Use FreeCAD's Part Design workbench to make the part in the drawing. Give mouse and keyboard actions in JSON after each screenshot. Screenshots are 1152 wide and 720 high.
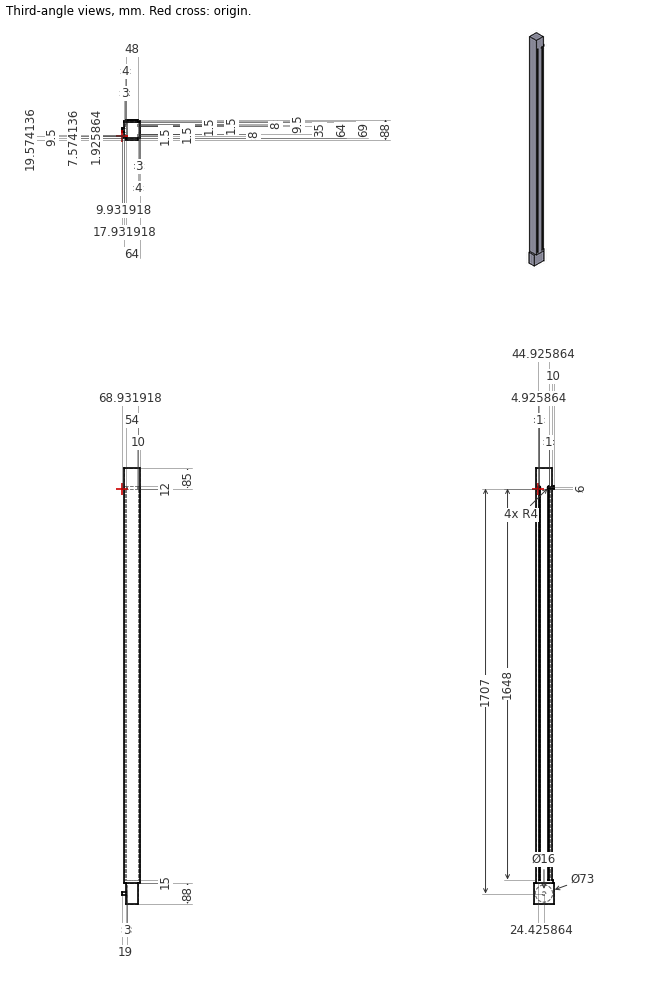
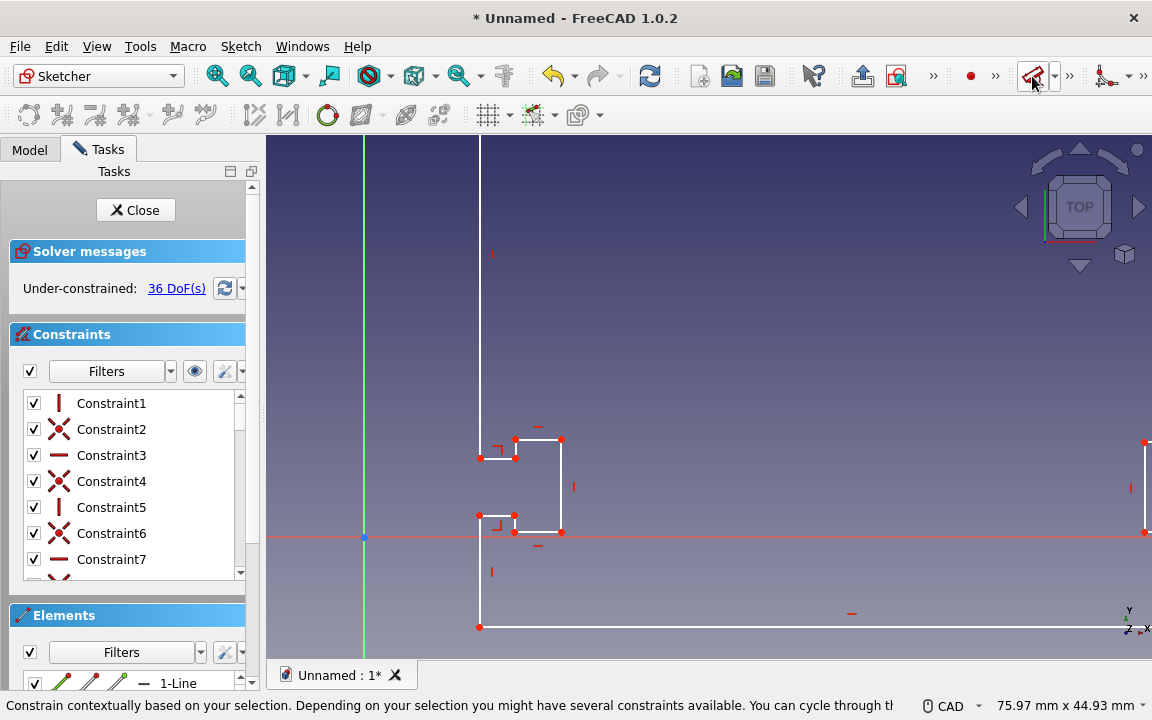
{"action": "scroll", "coordinate": [514, 515], "scroll_direction": "down", "scroll_amount": 4}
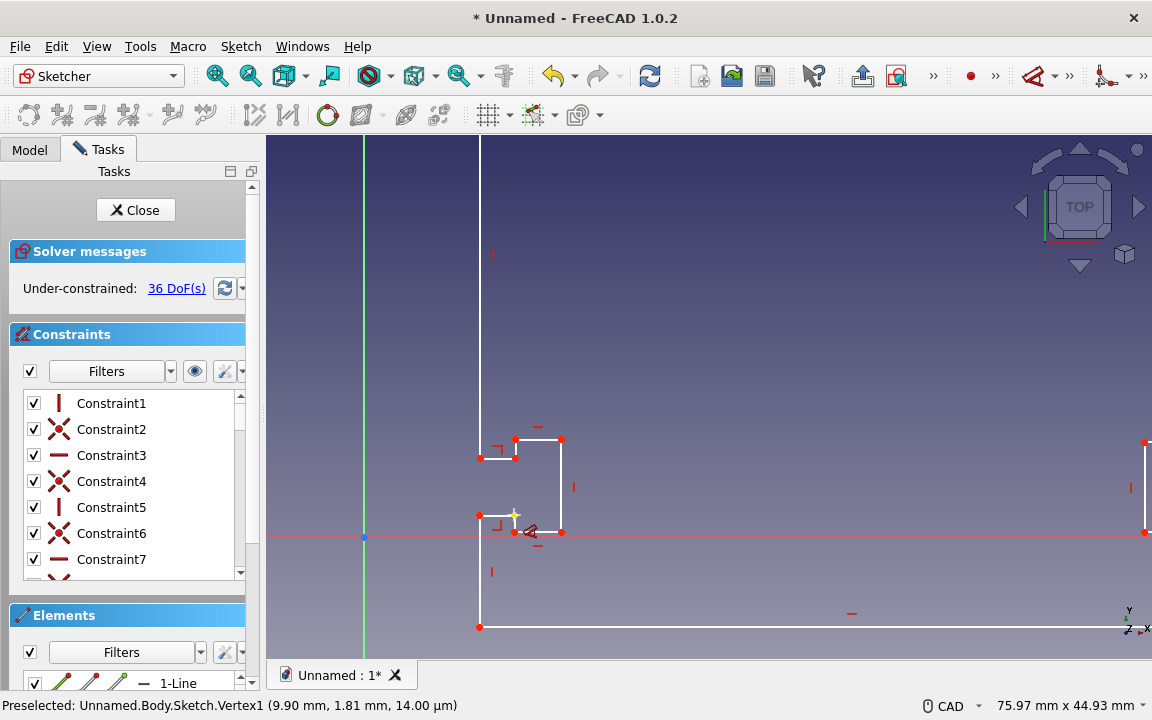
{"action": "scroll", "coordinate": [829, 516], "scroll_direction": "up", "scroll_amount": 6}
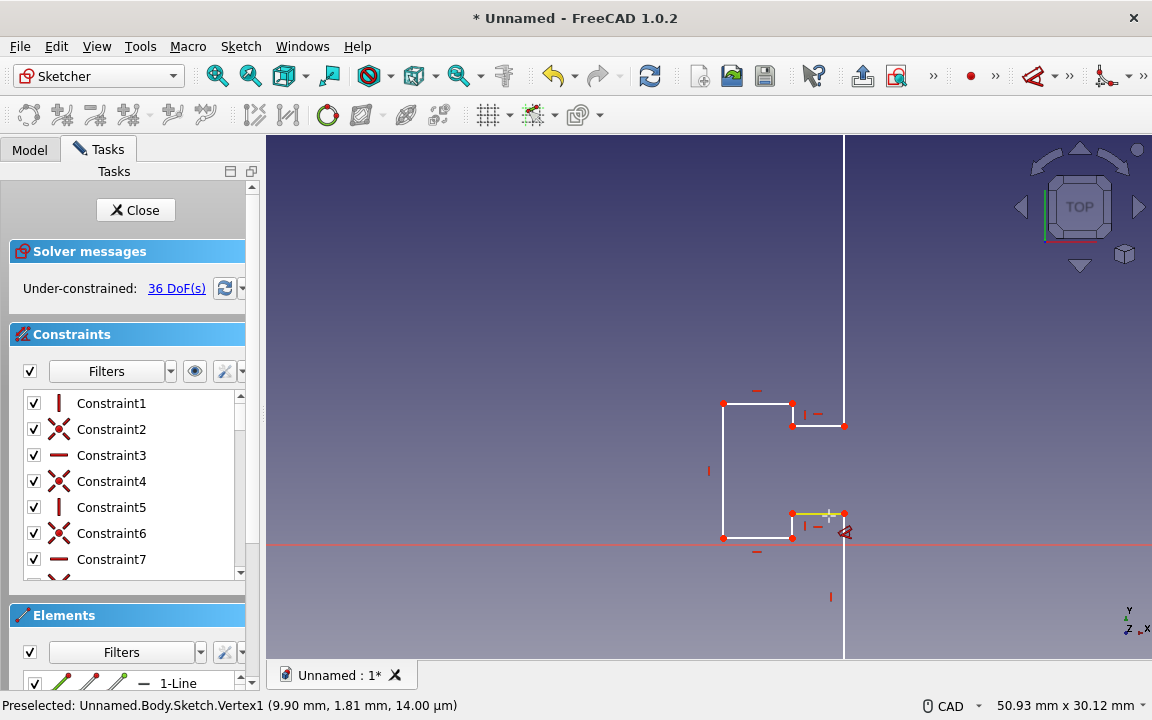
{"action": "left_click", "coordinate": [829, 514]}
{"action": "left_click", "coordinate": [818, 480]}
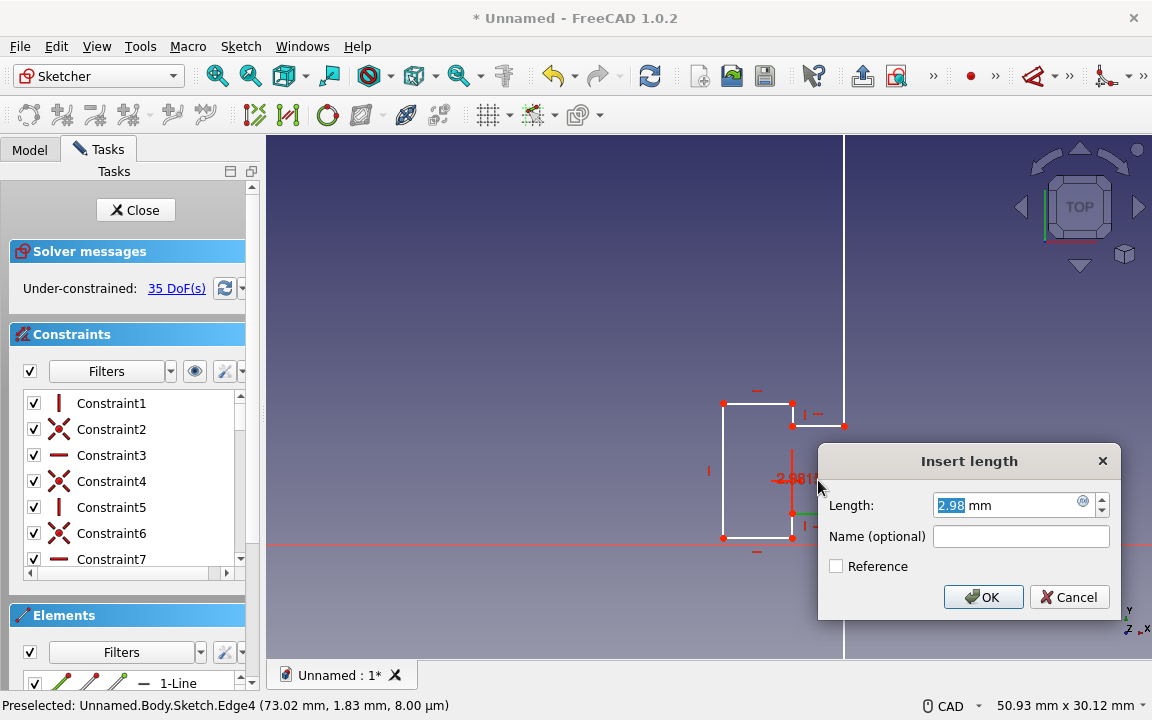
{"action": "type", "text": "3"}
{"action": "key", "text": "Return"}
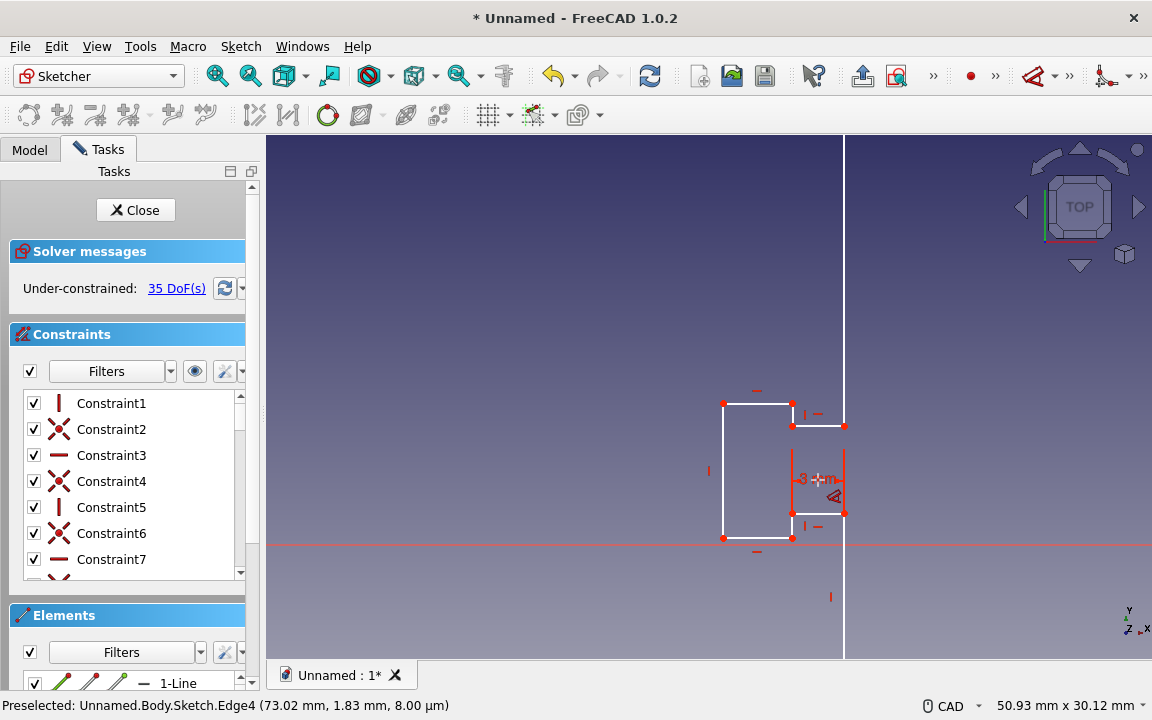
{"action": "scroll", "coordinate": [771, 538], "scroll_direction": "up", "scroll_amount": 4}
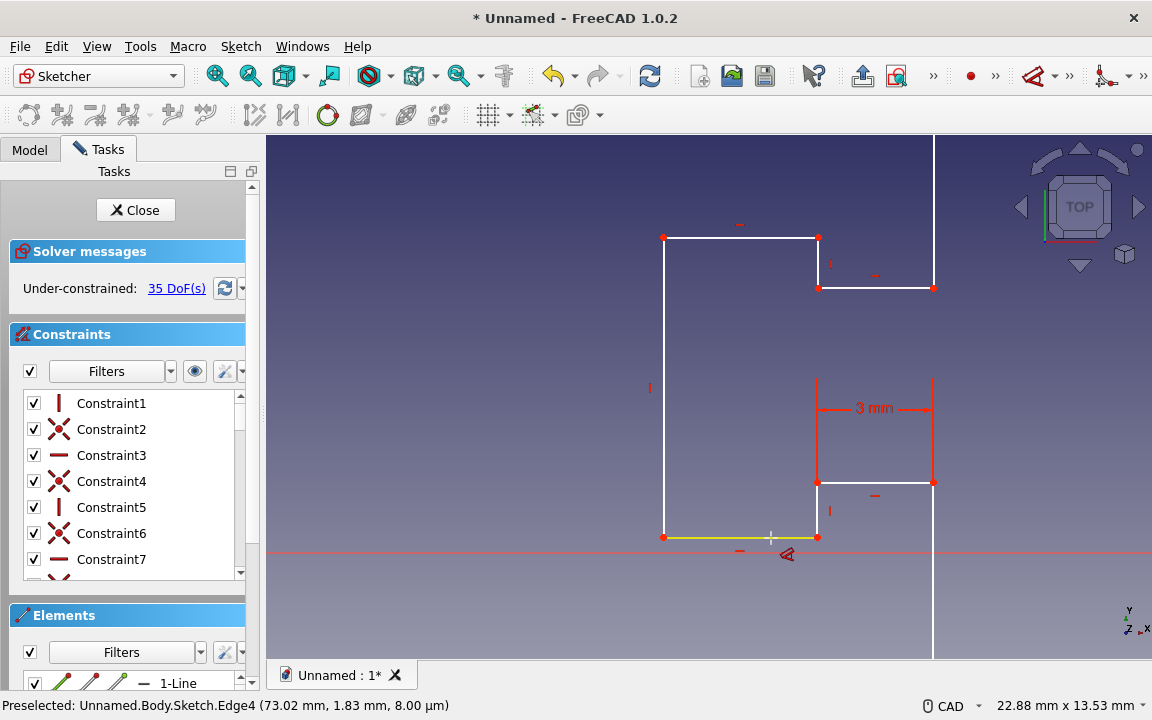
{"action": "left_click", "coordinate": [771, 538]}
{"action": "left_click", "coordinate": [740, 572]}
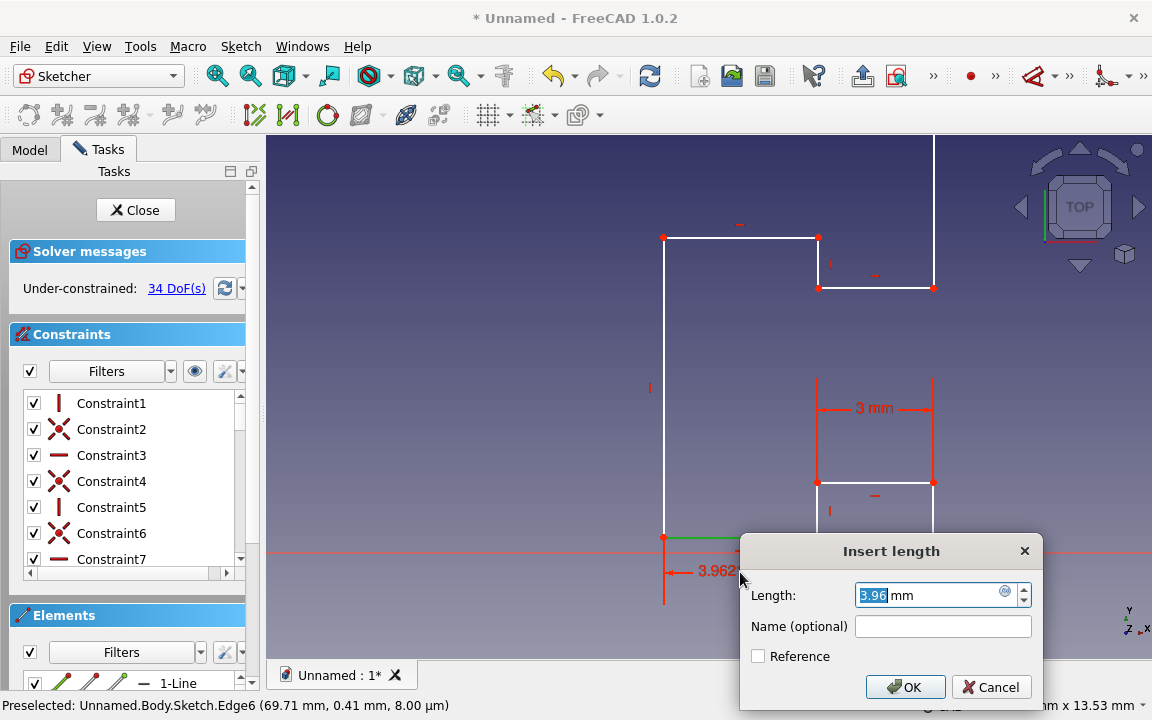
{"action": "type", "text": "4"}
{"action": "key", "text": "Return"}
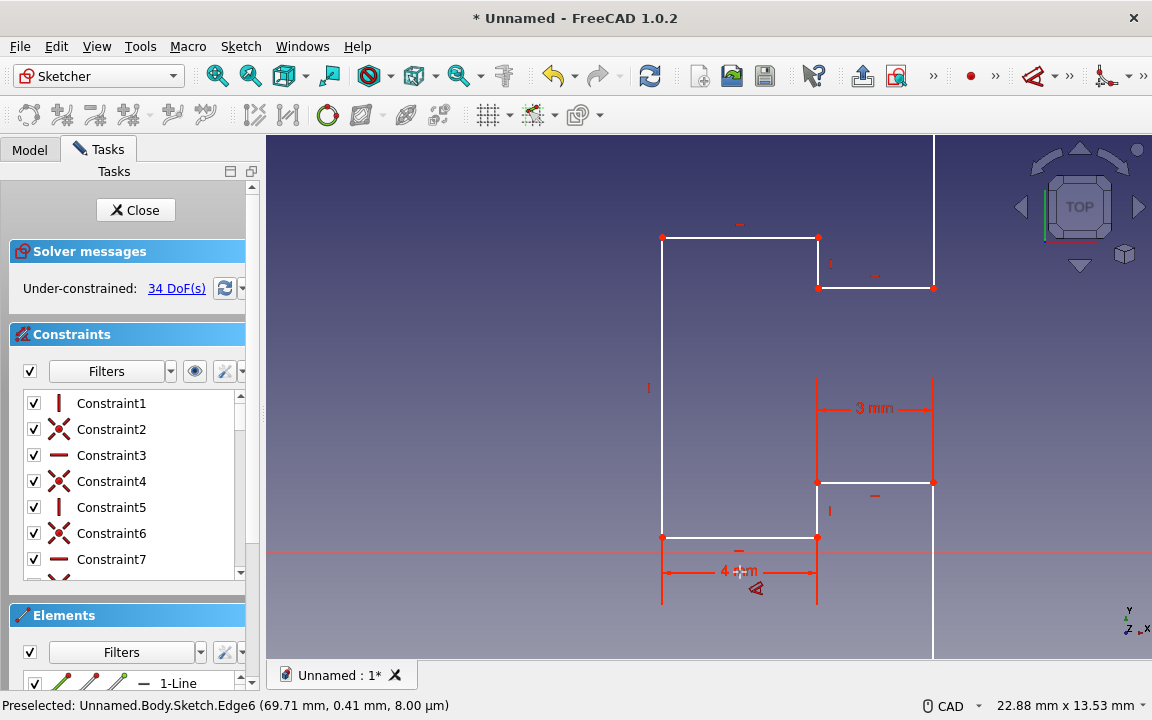
{"action": "scroll", "coordinate": [818, 521], "scroll_direction": "down", "scroll_amount": 10}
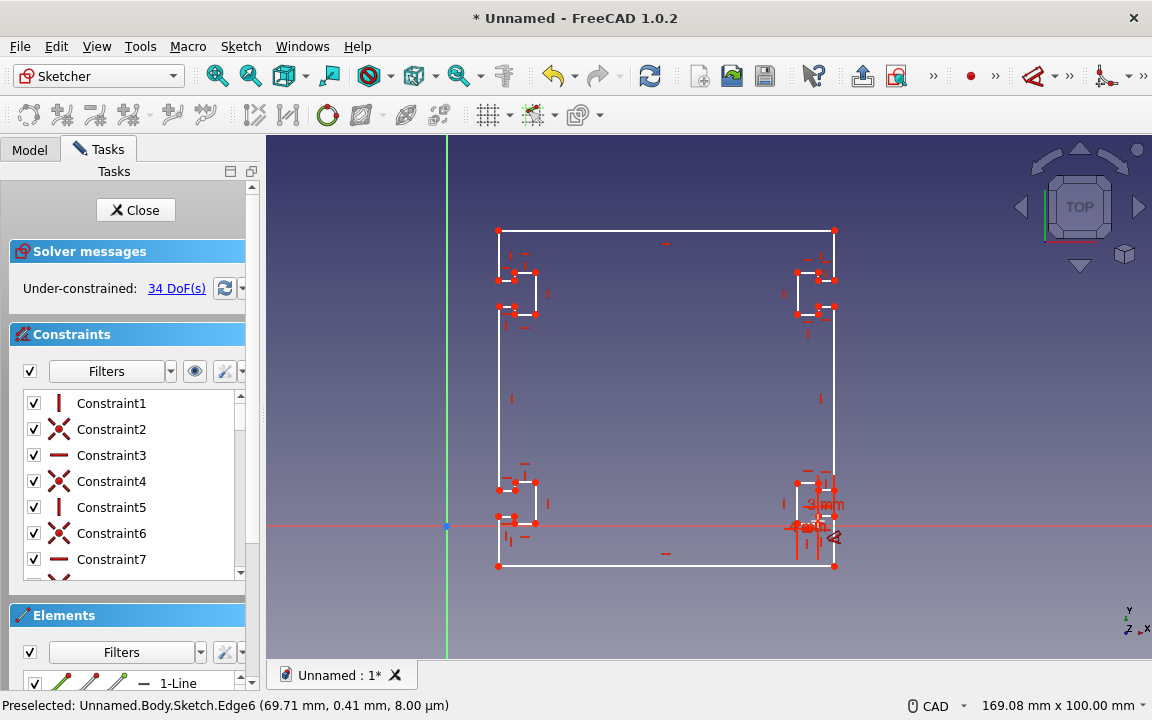
{"action": "left_click", "coordinate": [797, 512]}
{"action": "left_click", "coordinate": [739, 504]}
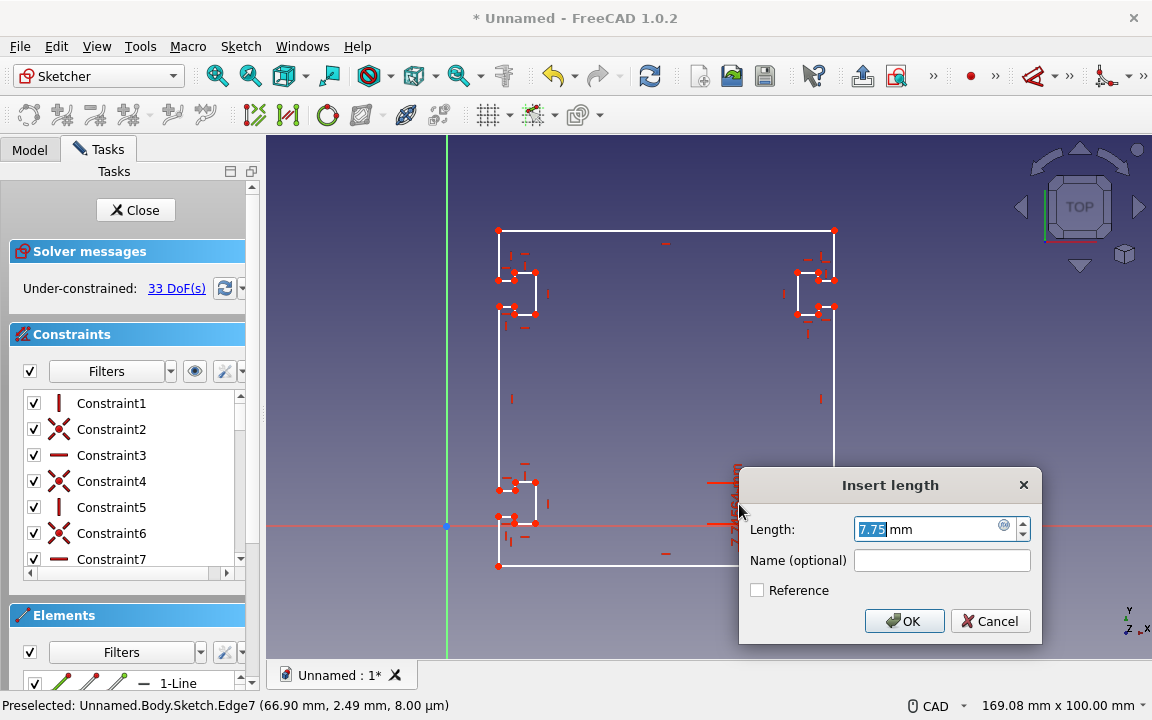
{"action": "type", "text": "8"}
{"action": "key", "text": "Return"}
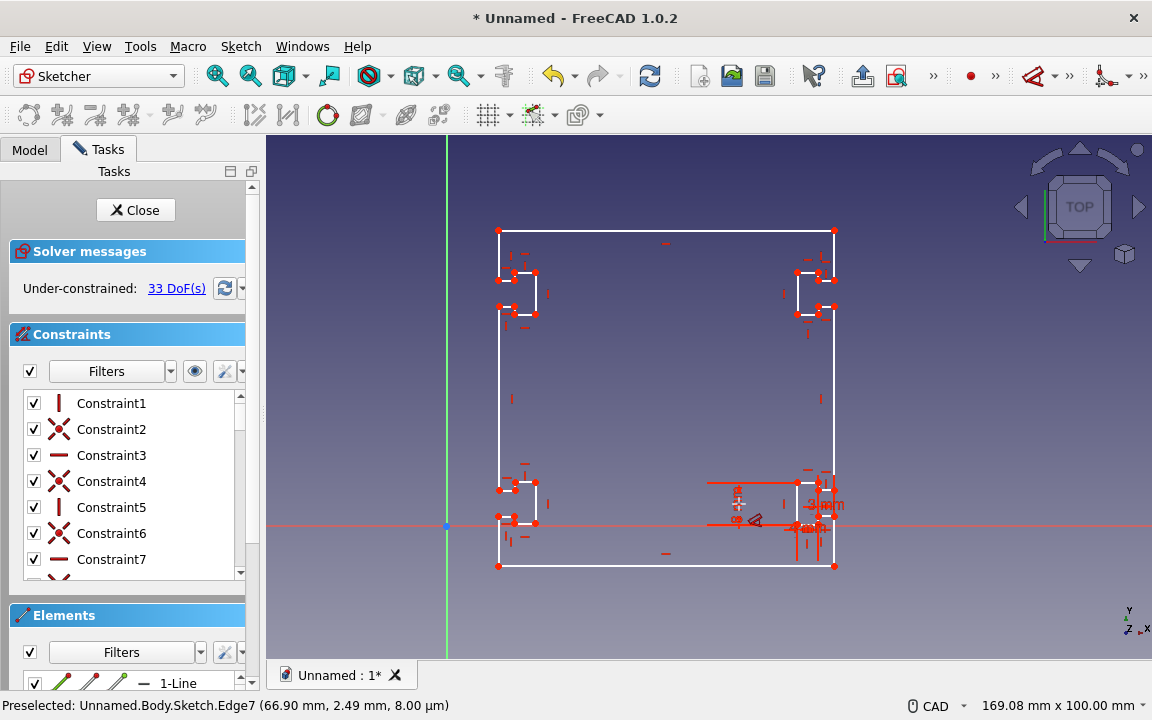
{"action": "scroll", "coordinate": [808, 483], "scroll_direction": "up", "scroll_amount": 4}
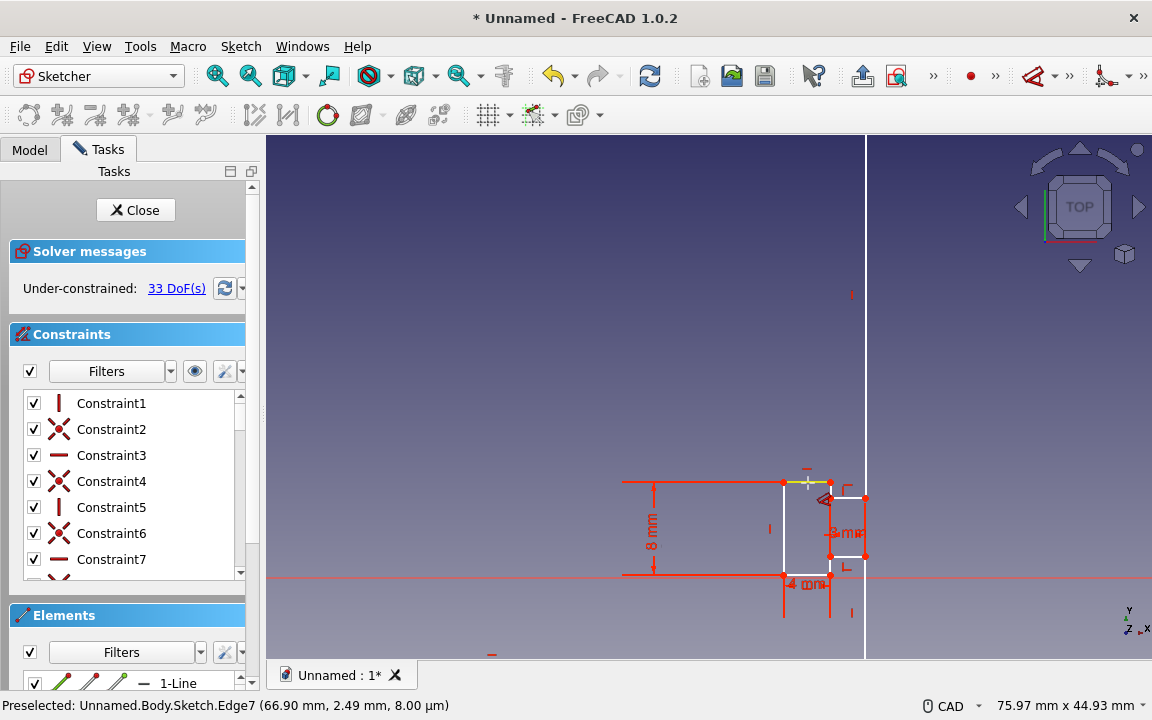
{"action": "left_click", "coordinate": [807, 482]}
{"action": "left_click", "coordinate": [807, 448]}